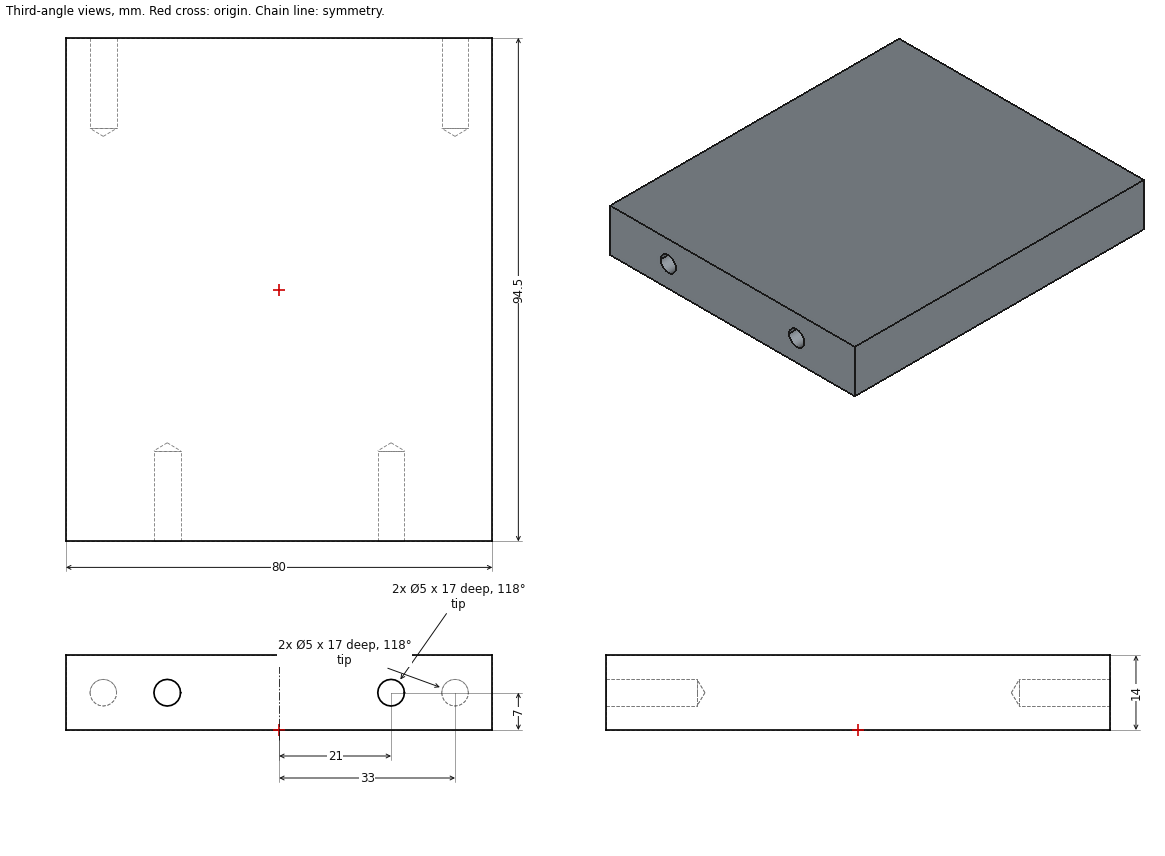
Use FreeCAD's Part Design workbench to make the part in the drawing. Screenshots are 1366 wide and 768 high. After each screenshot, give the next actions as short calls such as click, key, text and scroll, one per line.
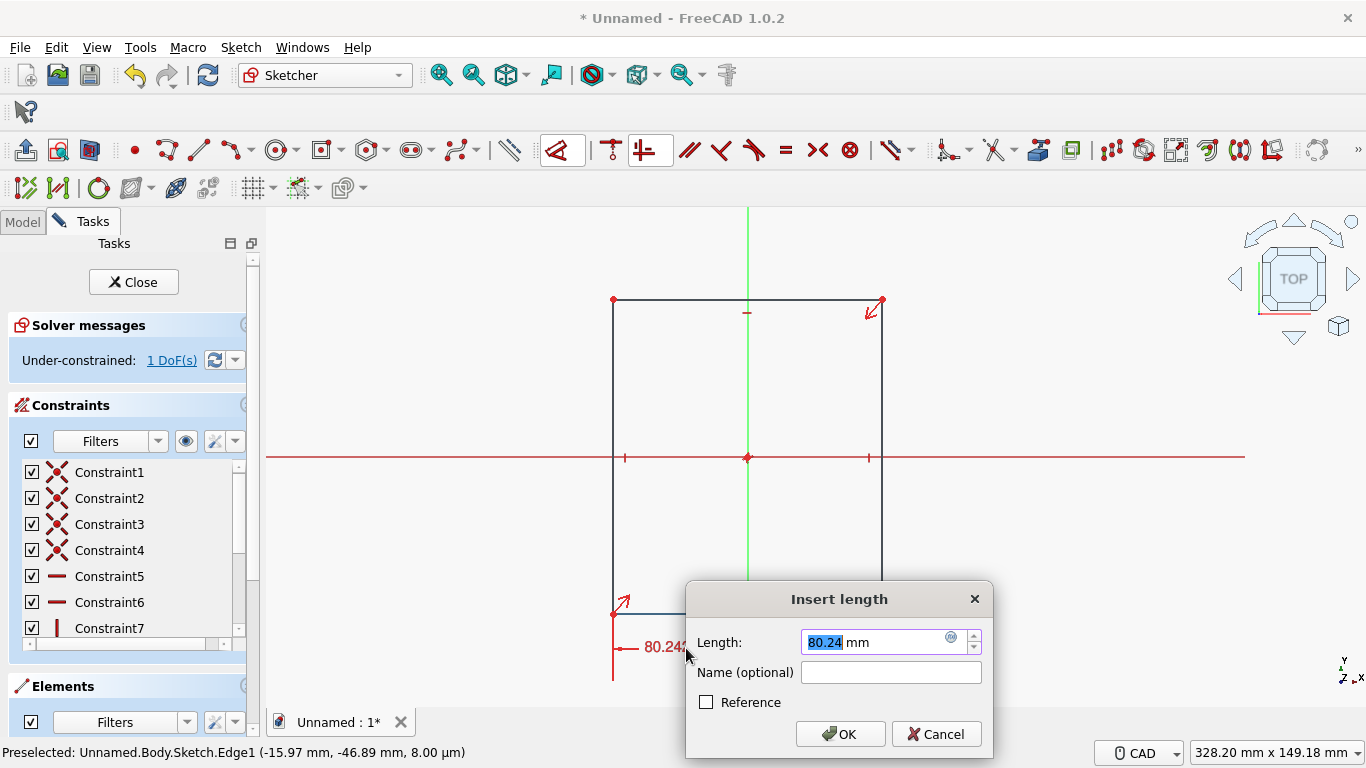
text(80)
key(Return)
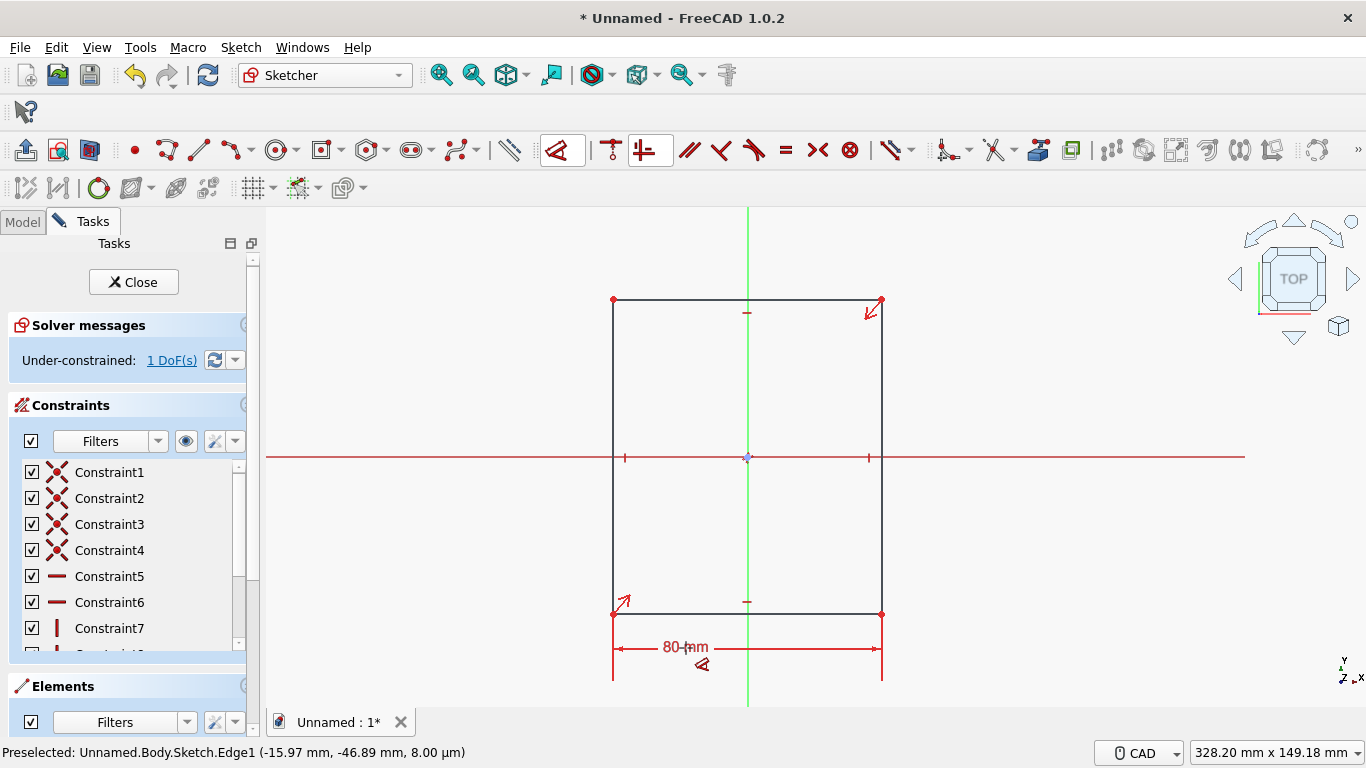
click(882, 520)
click(916, 385)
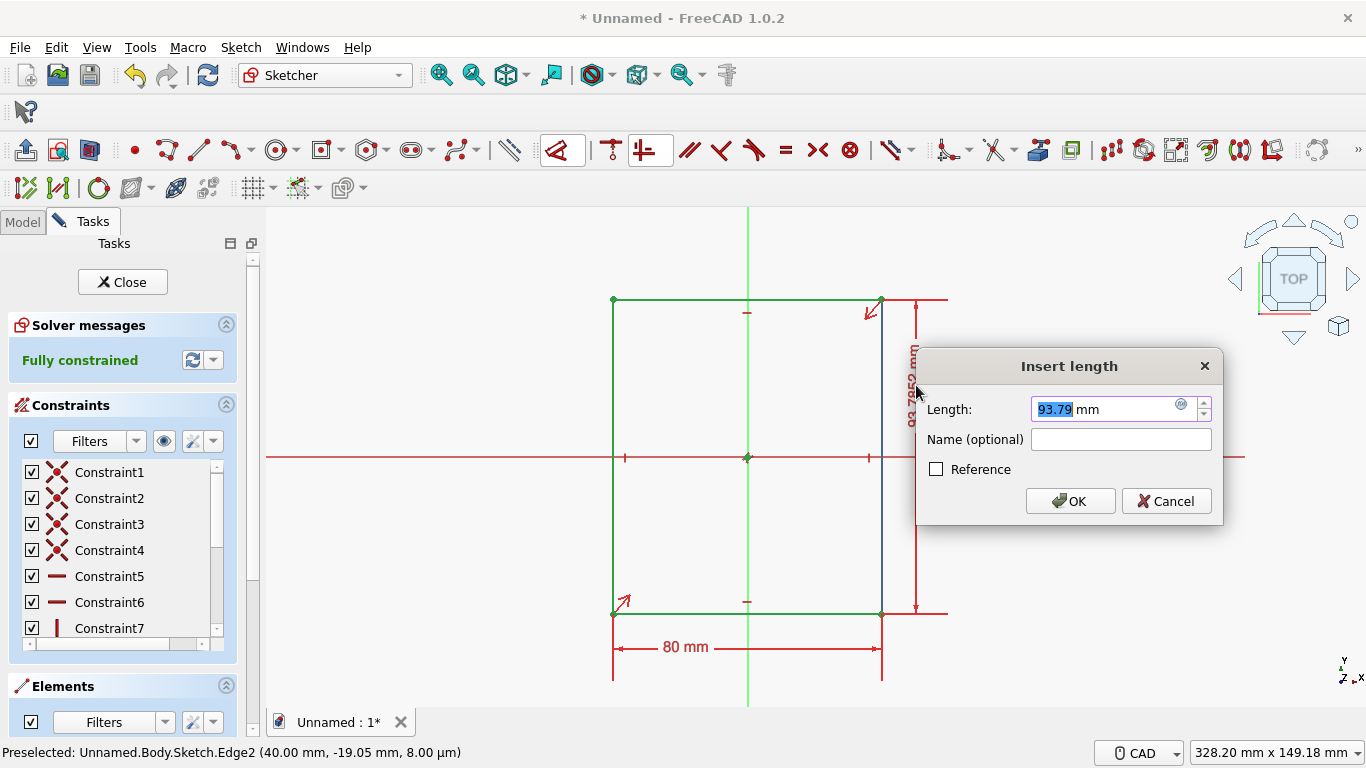
text(94.5)
key(Return)
key(Escape)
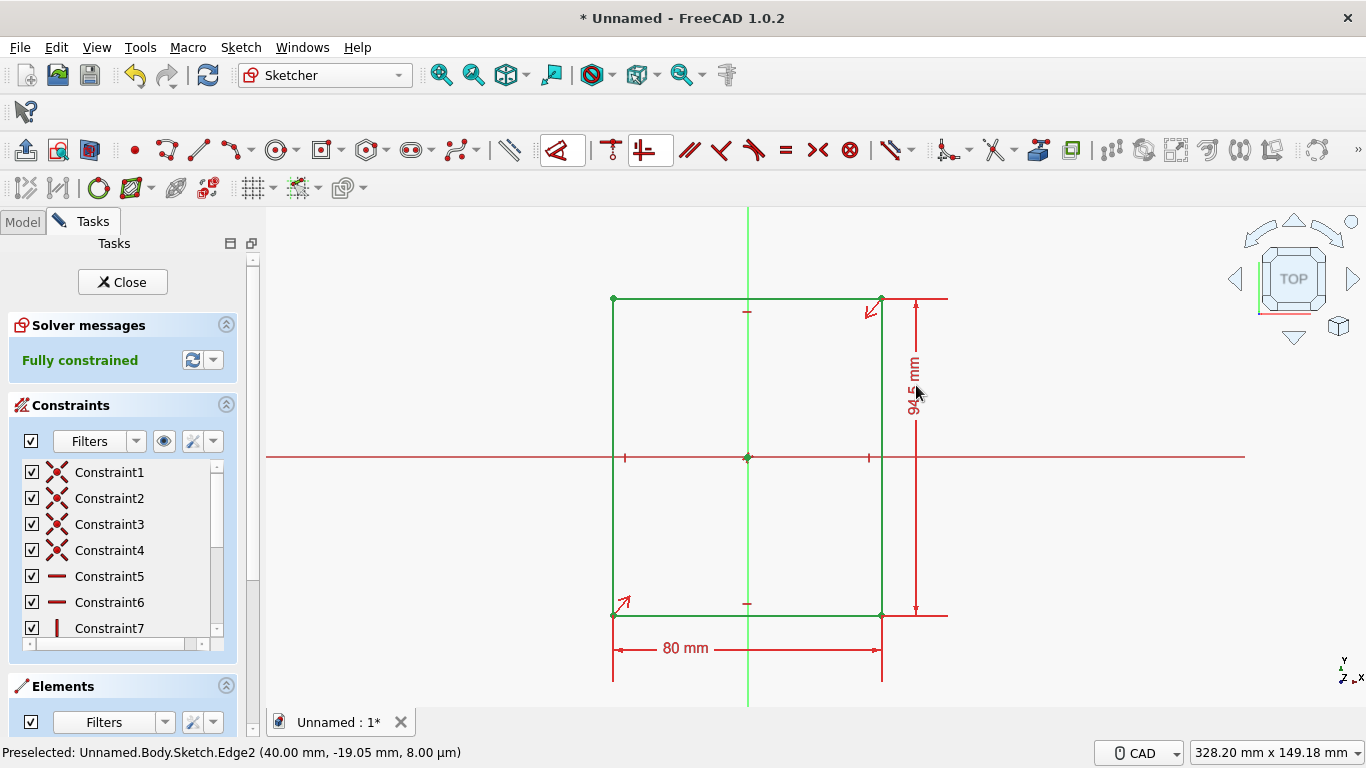
click(123, 282)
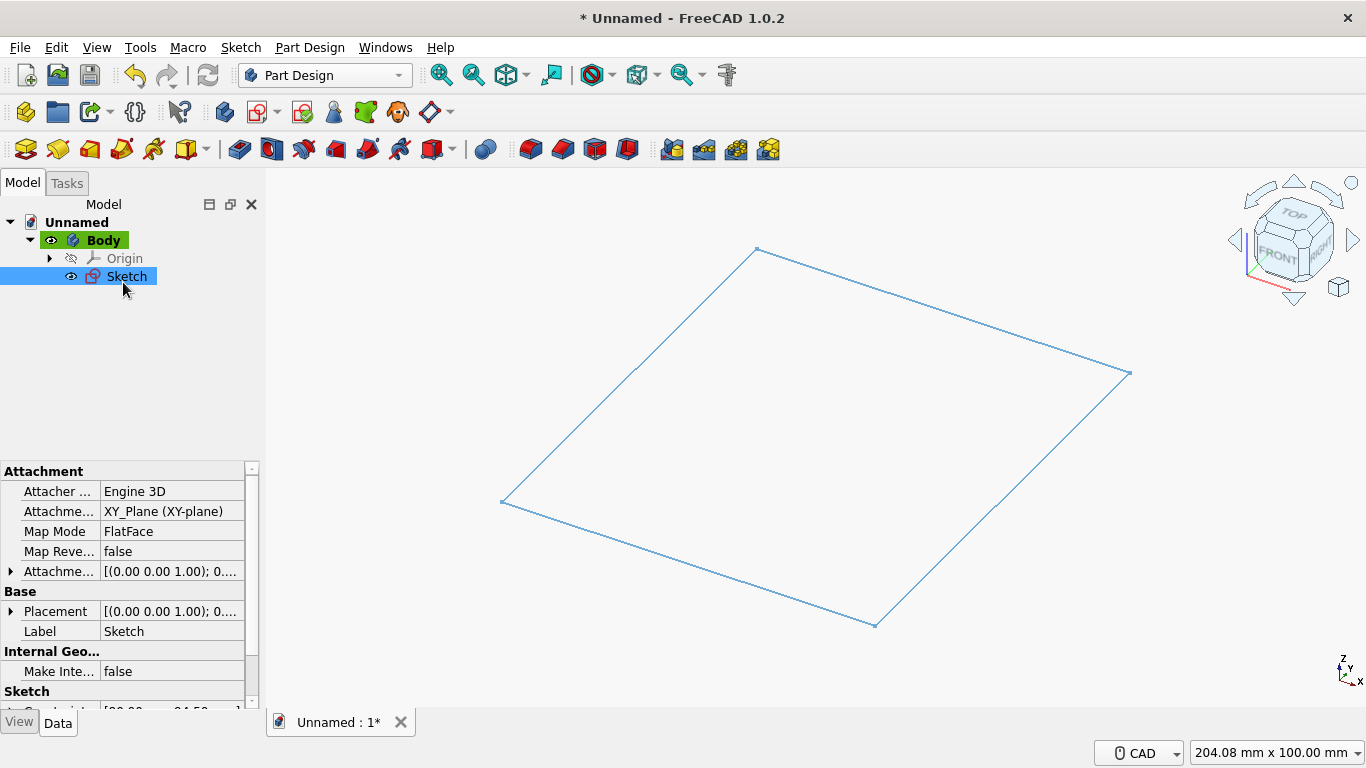
click(26, 150)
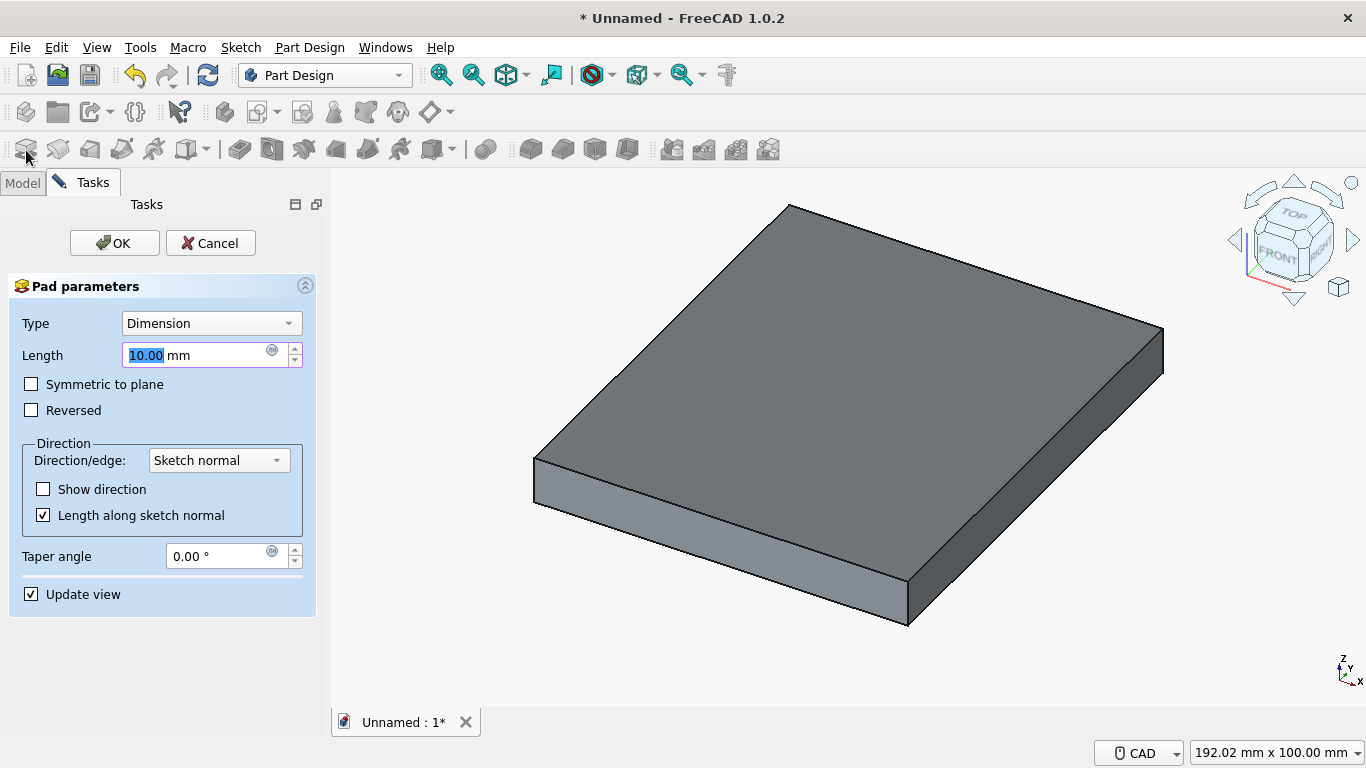
text(14)
key(Tab)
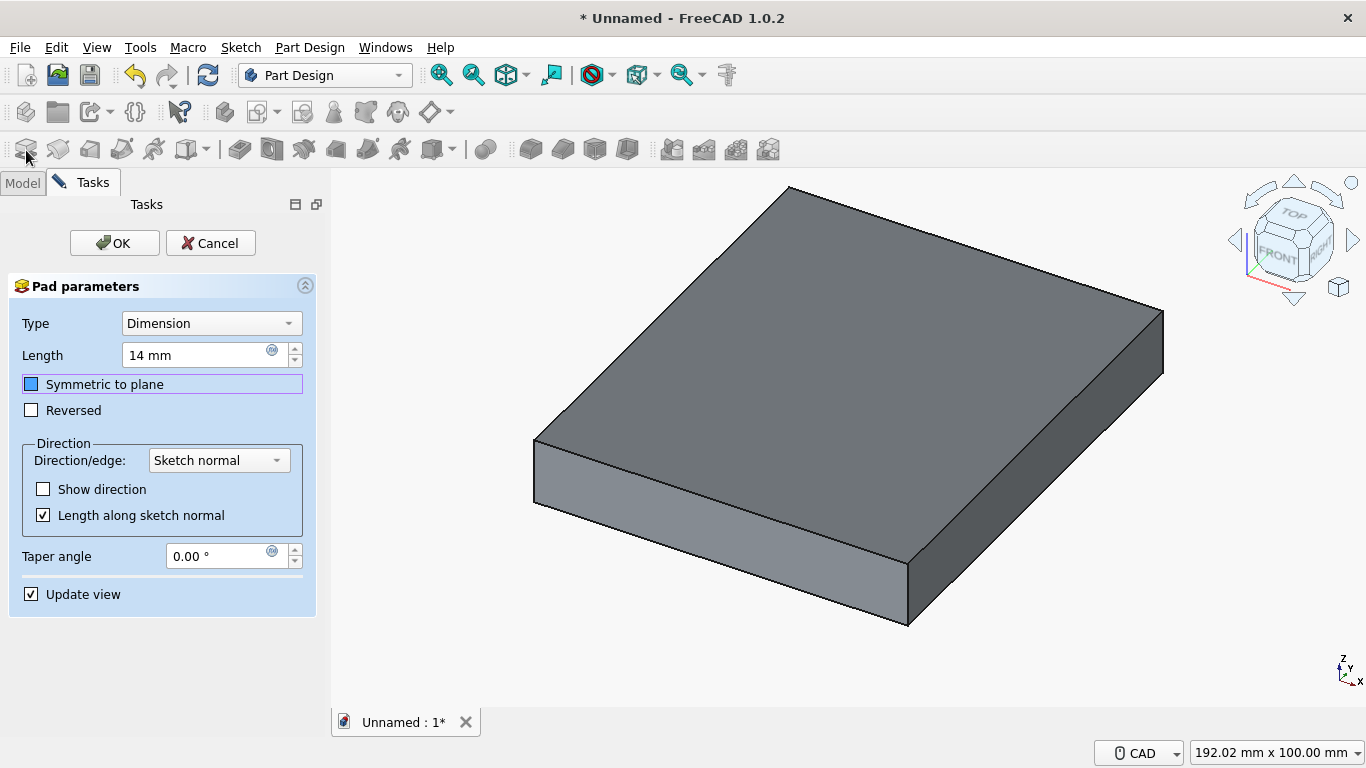
click(115, 243)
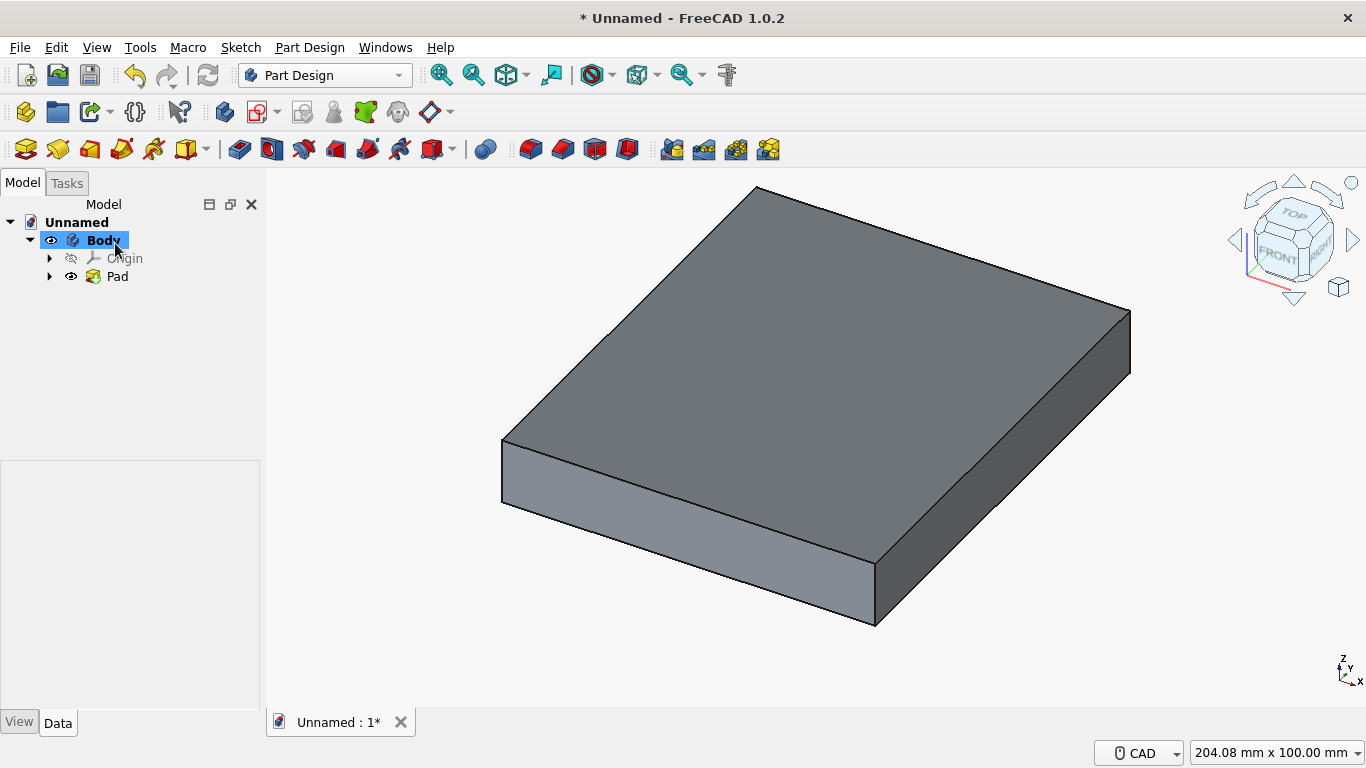
click(795, 567)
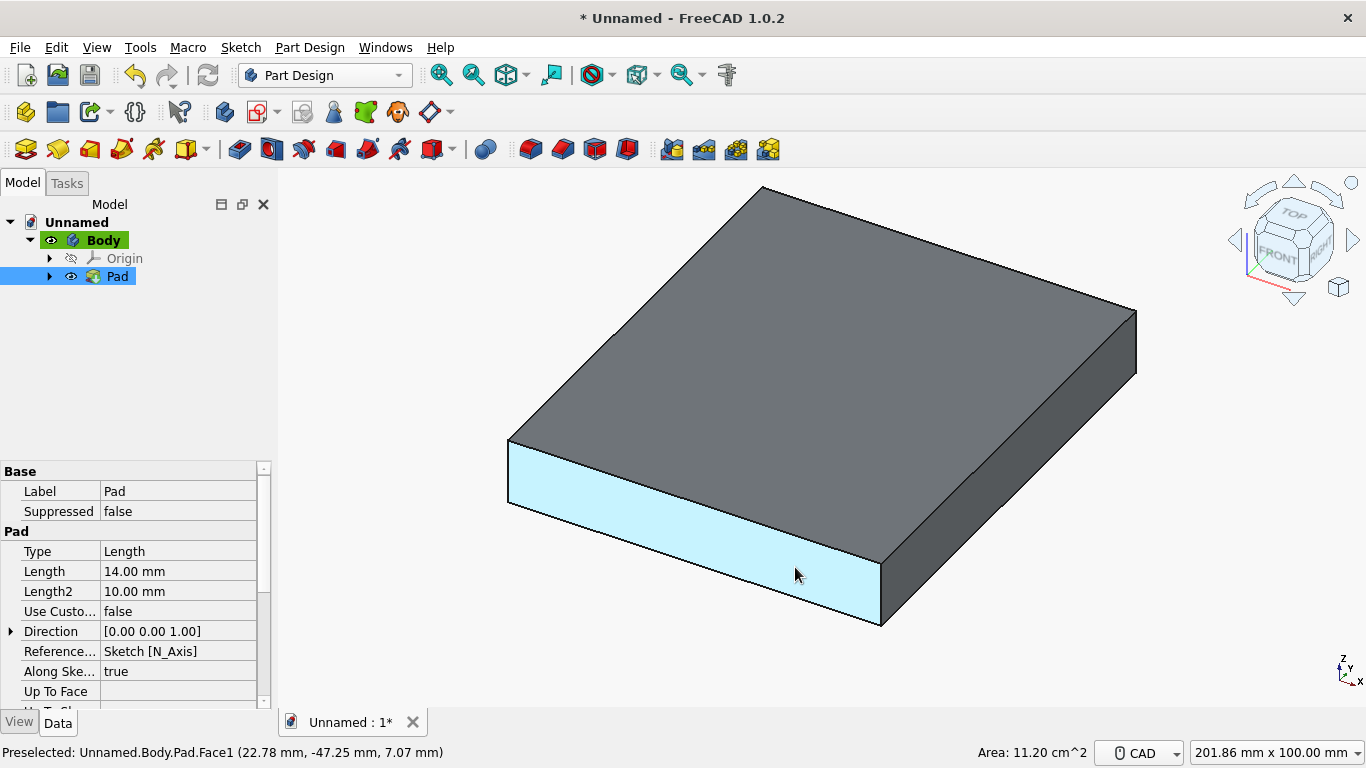
click(258, 112)